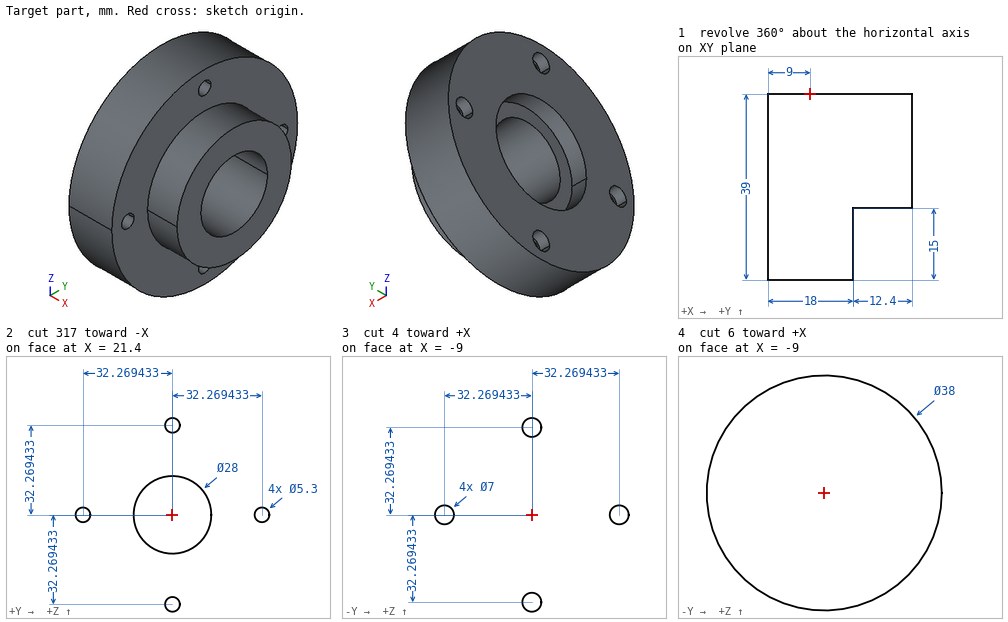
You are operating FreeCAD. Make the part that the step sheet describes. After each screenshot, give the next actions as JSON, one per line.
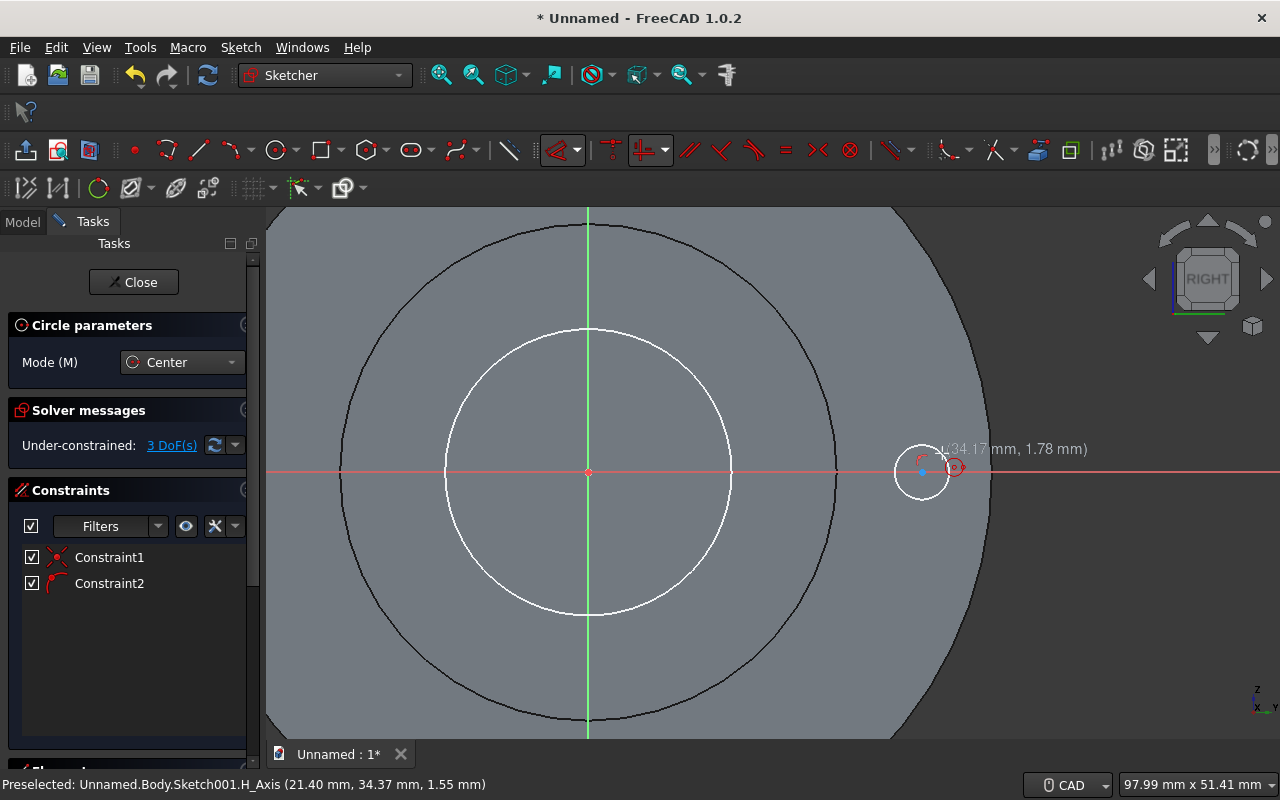
{"action": "scroll", "coordinate": [799, 474], "scroll_direction": "down", "scroll_amount": 4}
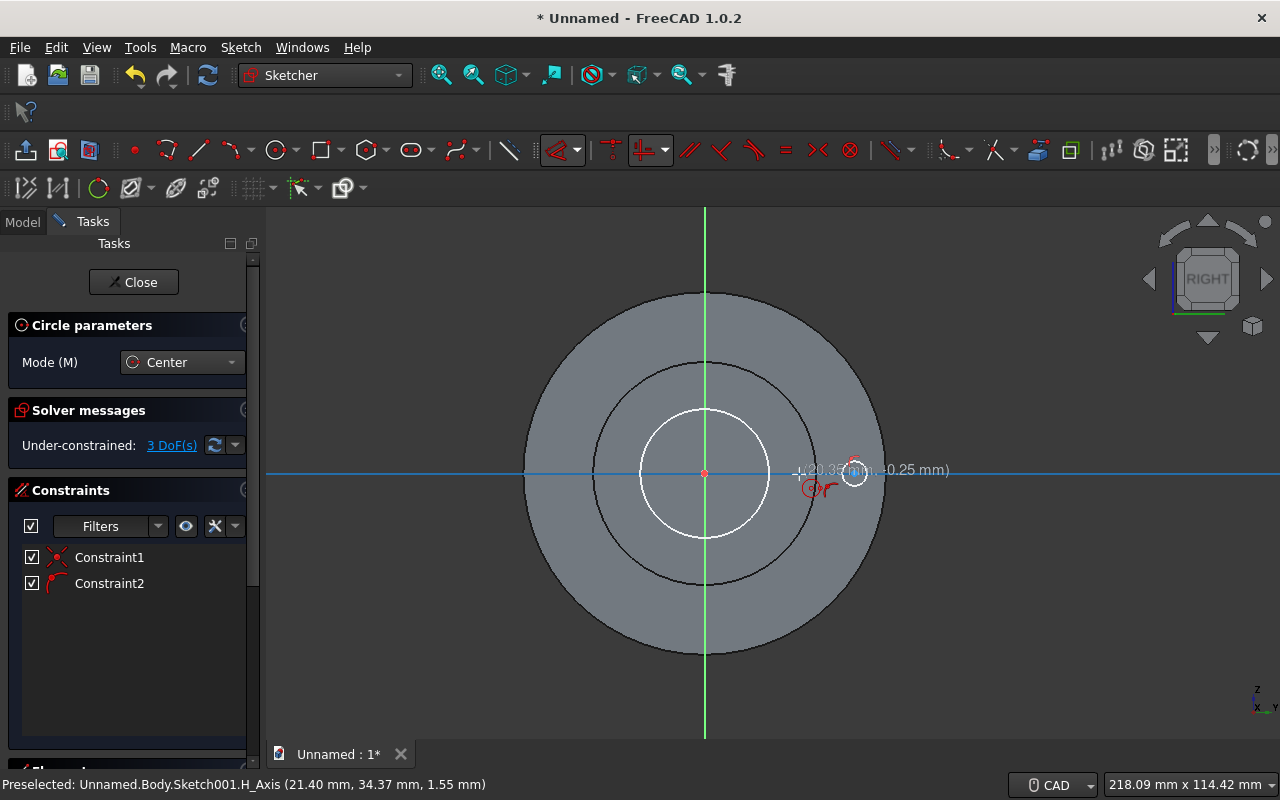
{"action": "scroll", "coordinate": [705, 624], "scroll_direction": "up", "scroll_amount": 4}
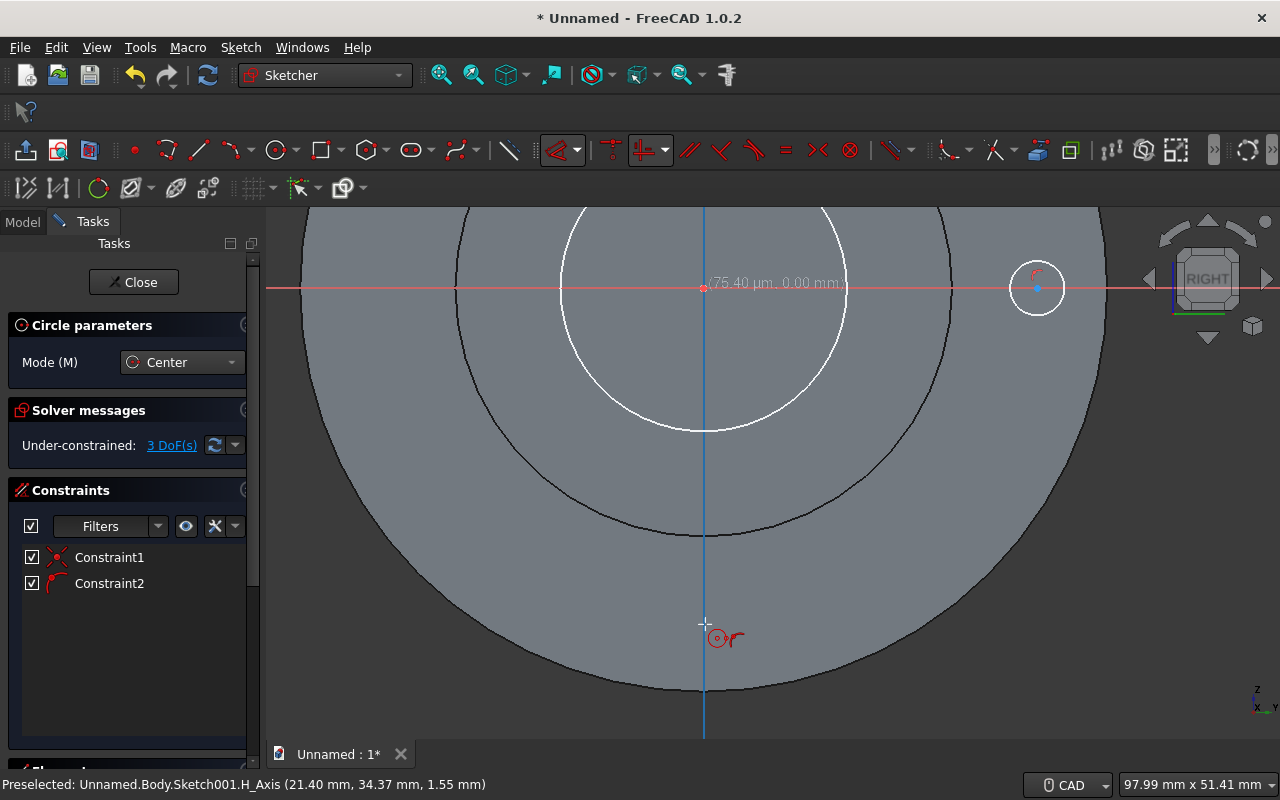
{"action": "left_click", "coordinate": [704, 622]}
{"action": "left_click", "coordinate": [723, 603]}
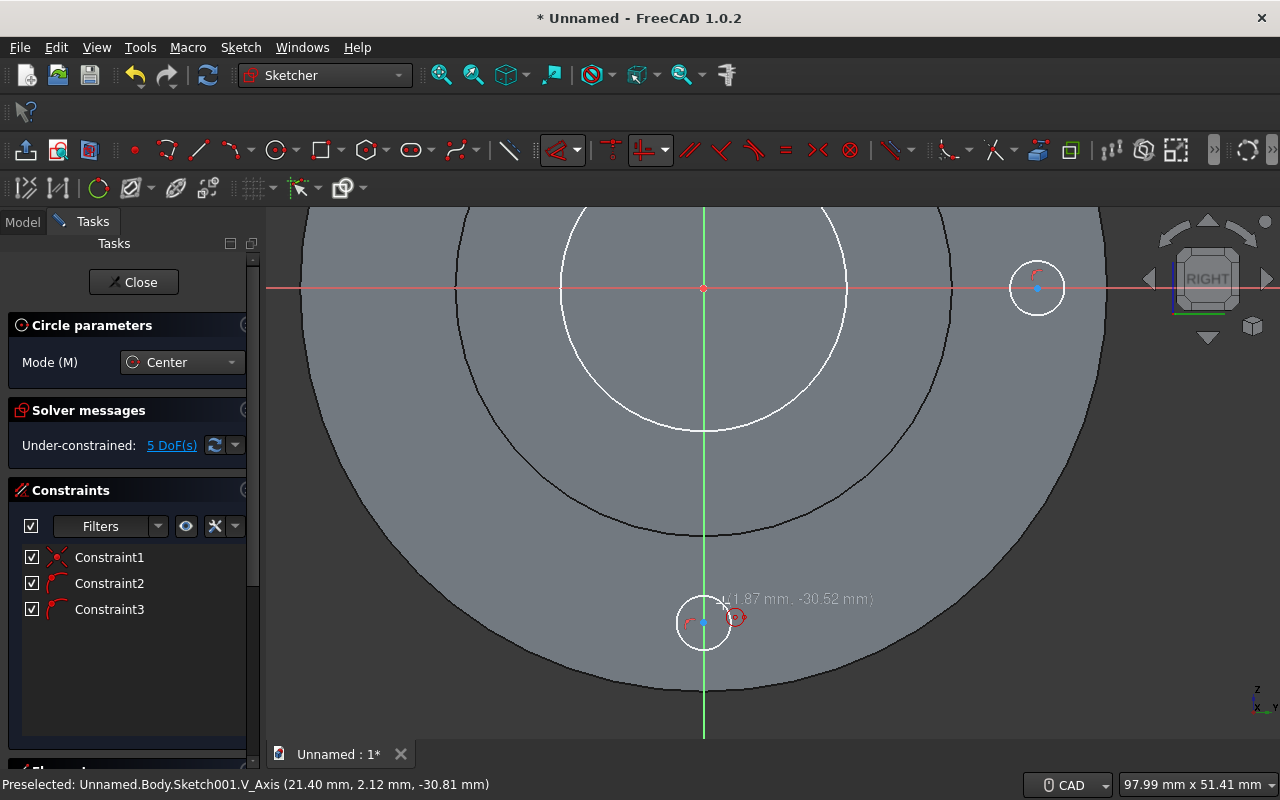
{"action": "left_click", "coordinate": [370, 288]}
{"action": "left_click", "coordinate": [389, 269]}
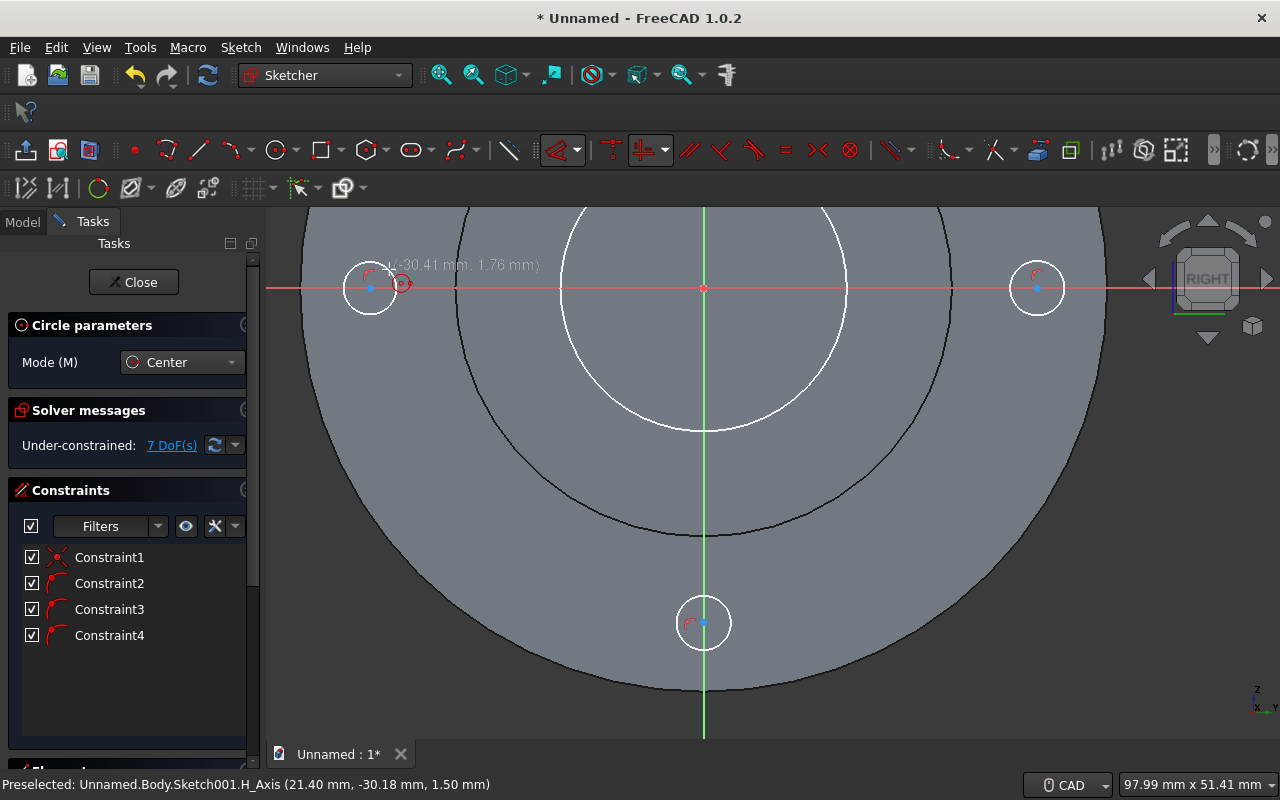
{"action": "scroll", "coordinate": [705, 624], "scroll_direction": "down", "scroll_amount": 4}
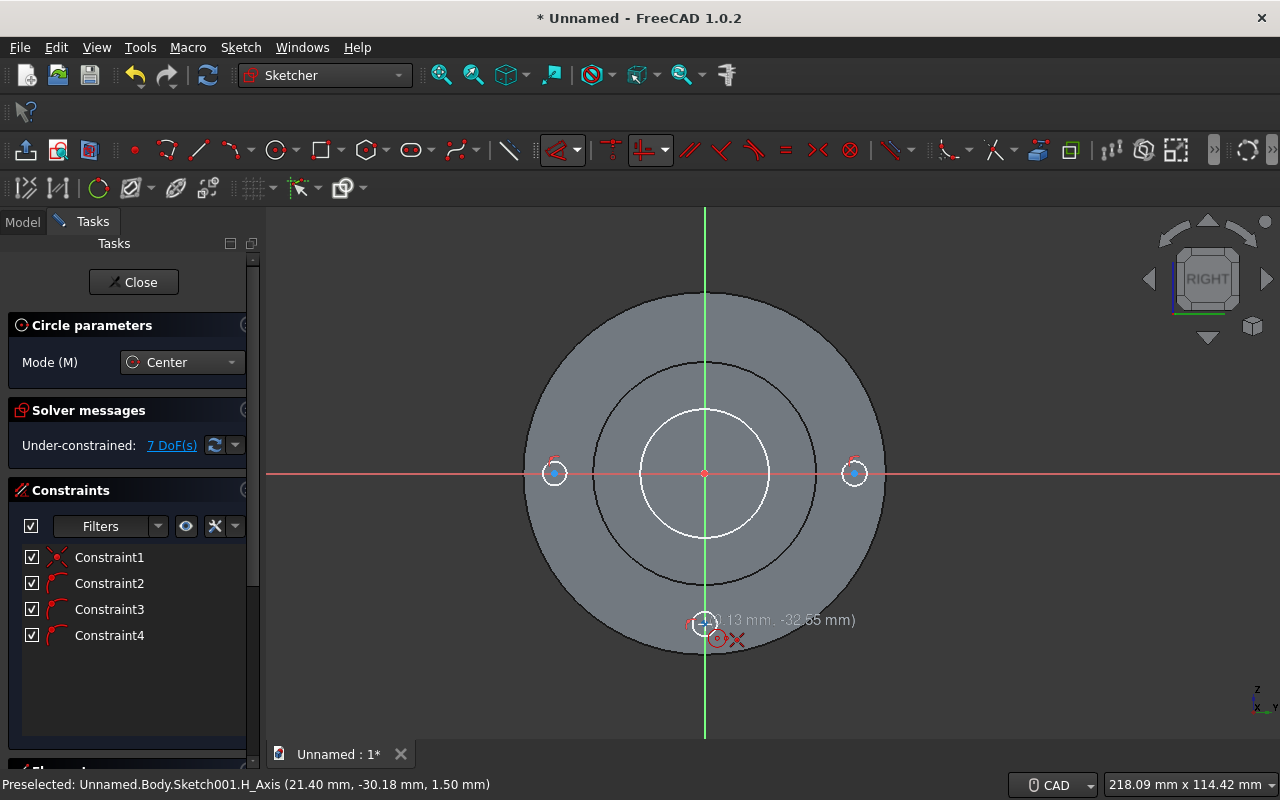
{"action": "scroll", "coordinate": [705, 324], "scroll_direction": "up", "scroll_amount": 4}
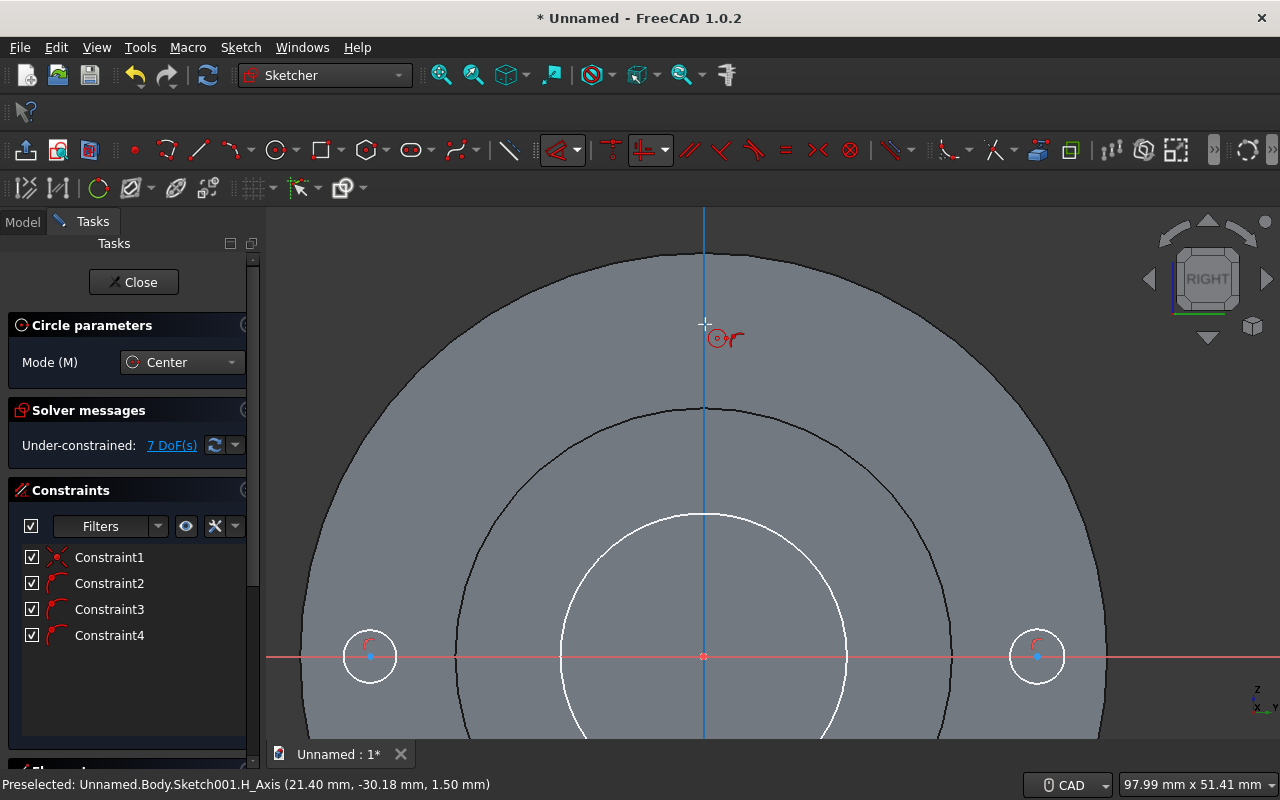
{"action": "left_click", "coordinate": [704, 323]}
{"action": "left_click", "coordinate": [723, 303]}
{"action": "key", "text": "Escape"}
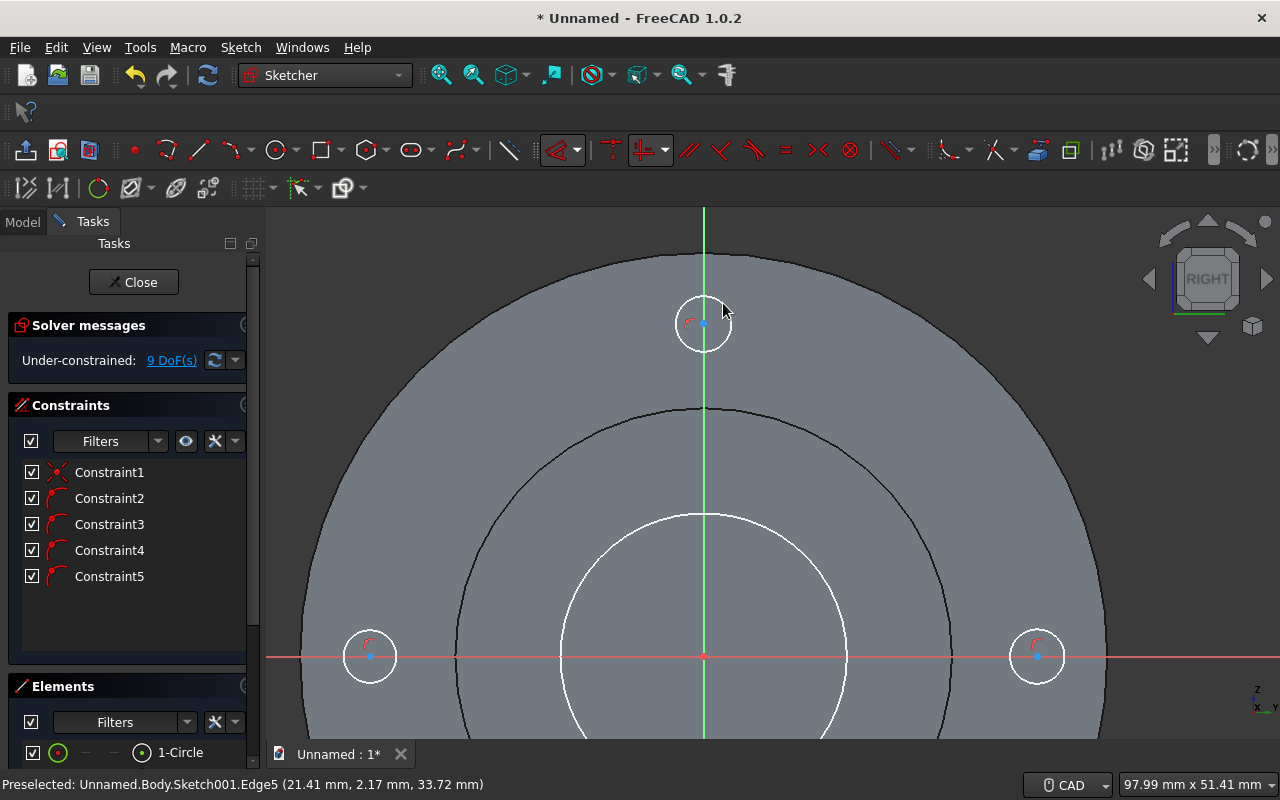
{"action": "left_click", "coordinate": [1056, 637]}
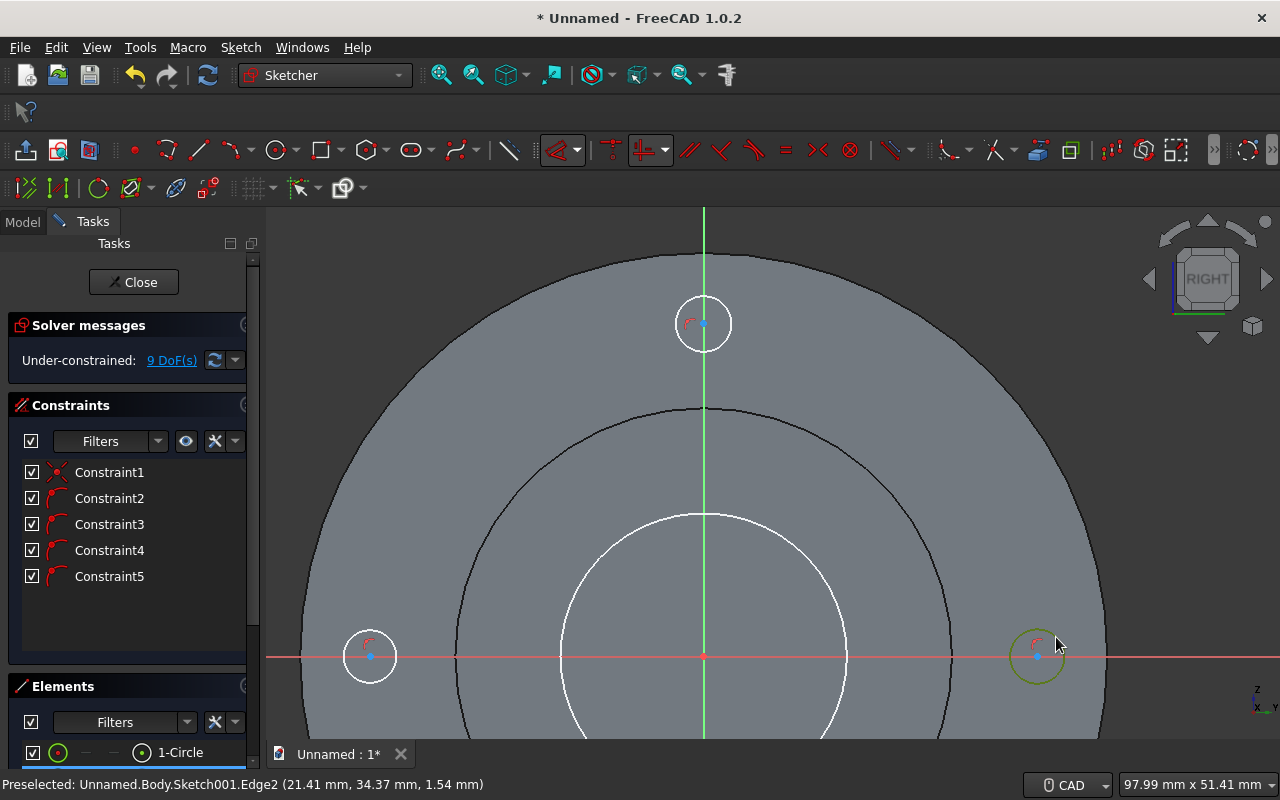
{"action": "scroll", "coordinate": [705, 323], "scroll_direction": "down", "scroll_amount": 4}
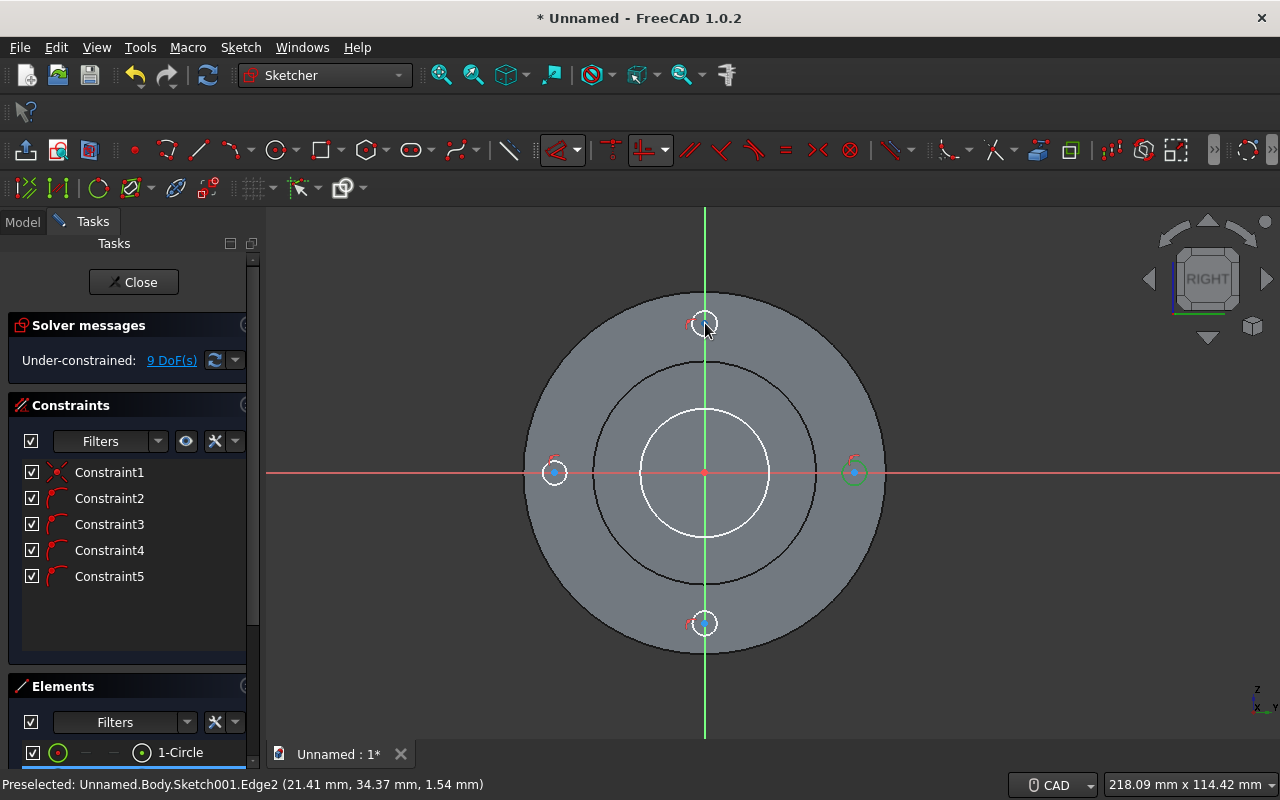
{"action": "scroll", "coordinate": [713, 615], "scroll_direction": "up", "scroll_amount": 3}